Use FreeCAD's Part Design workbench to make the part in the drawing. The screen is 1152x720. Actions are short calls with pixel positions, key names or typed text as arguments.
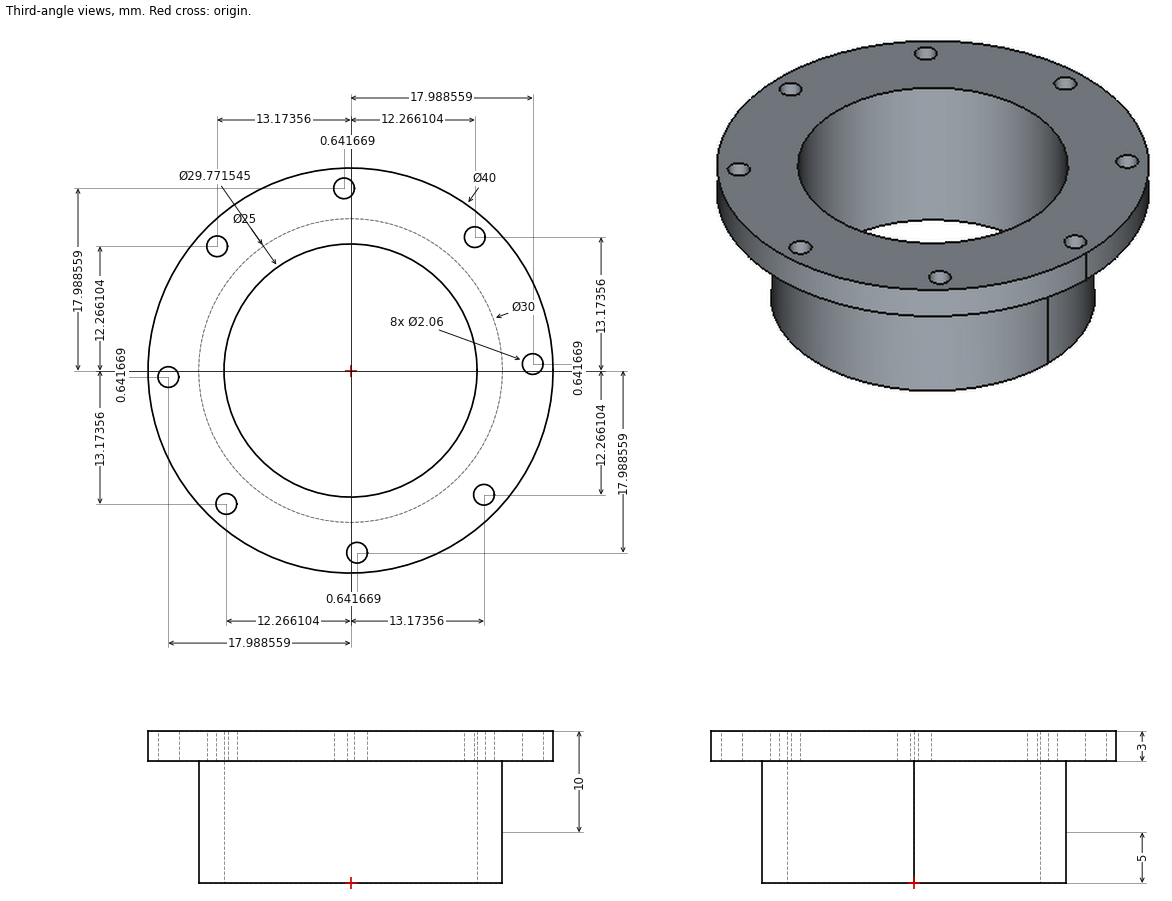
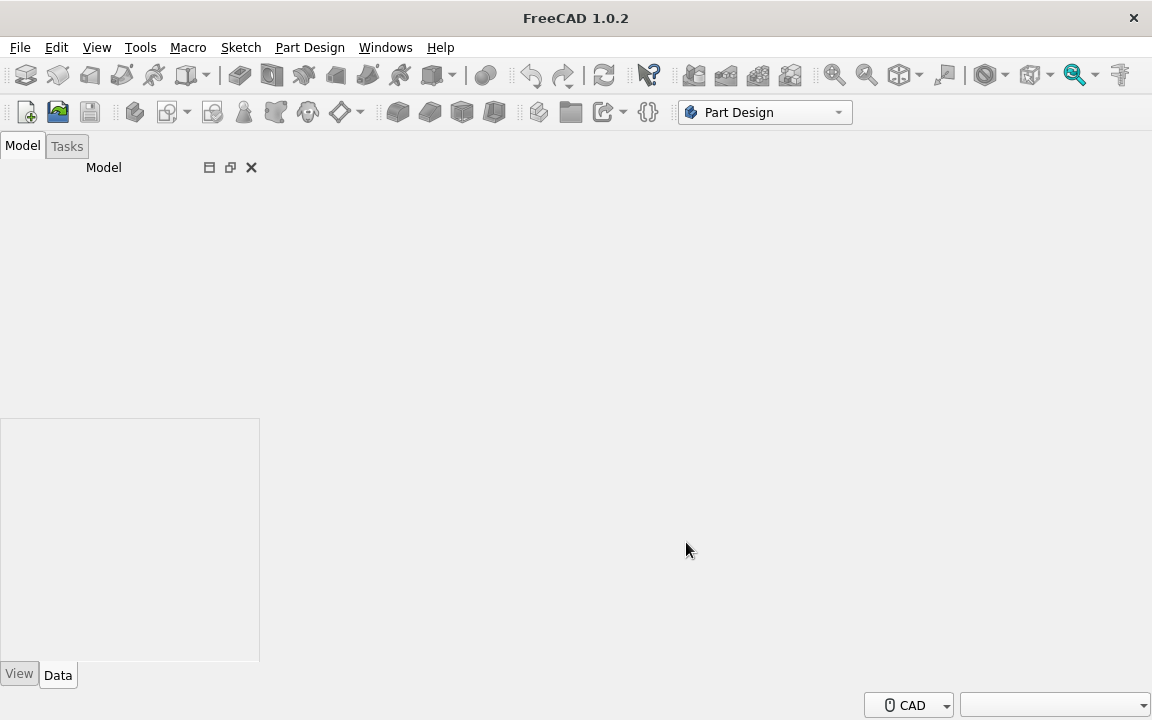
key(ctrl+n)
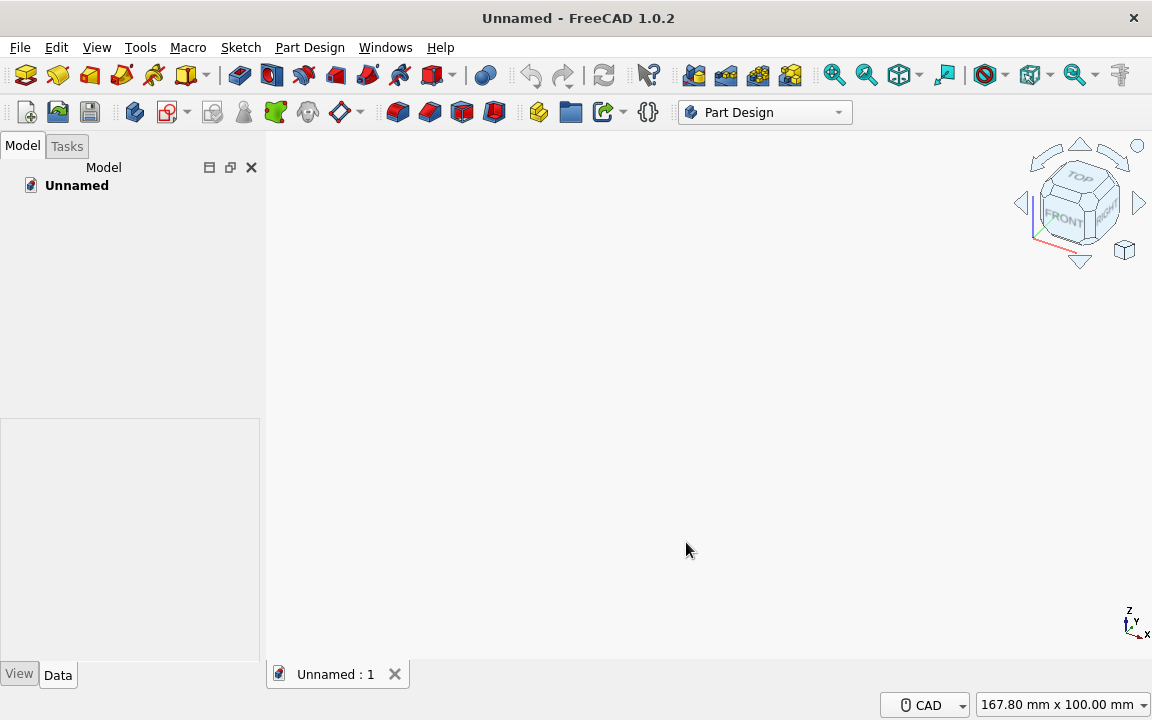
click(168, 112)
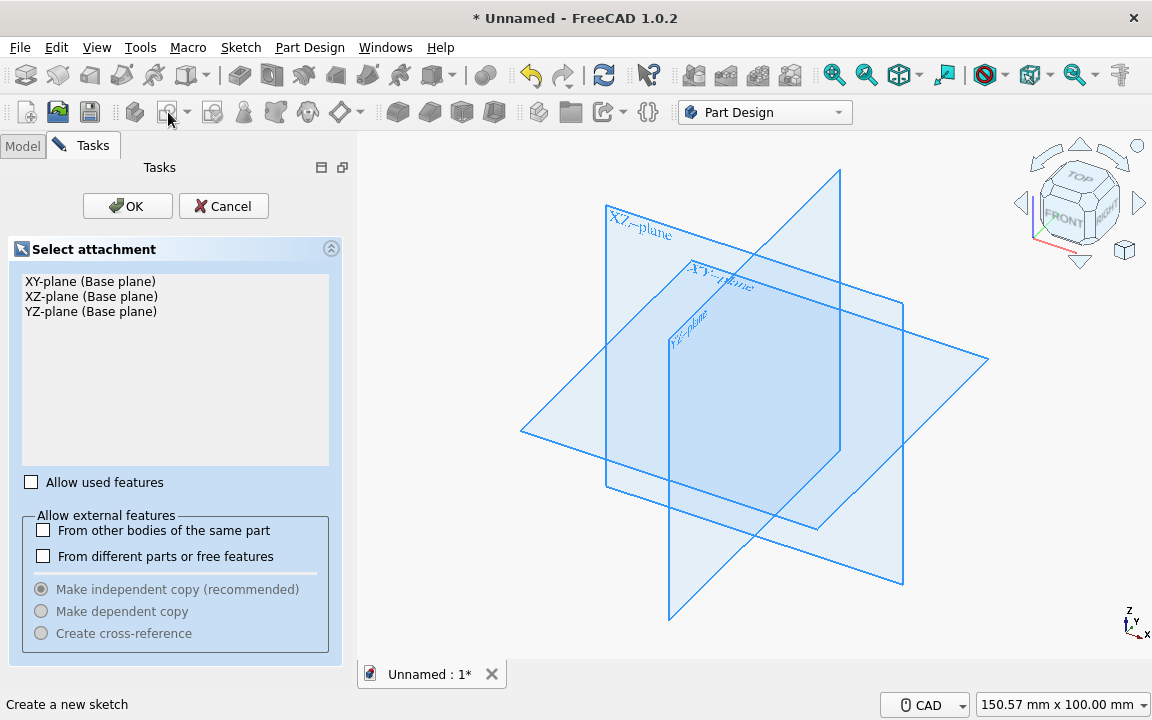
click(82, 282)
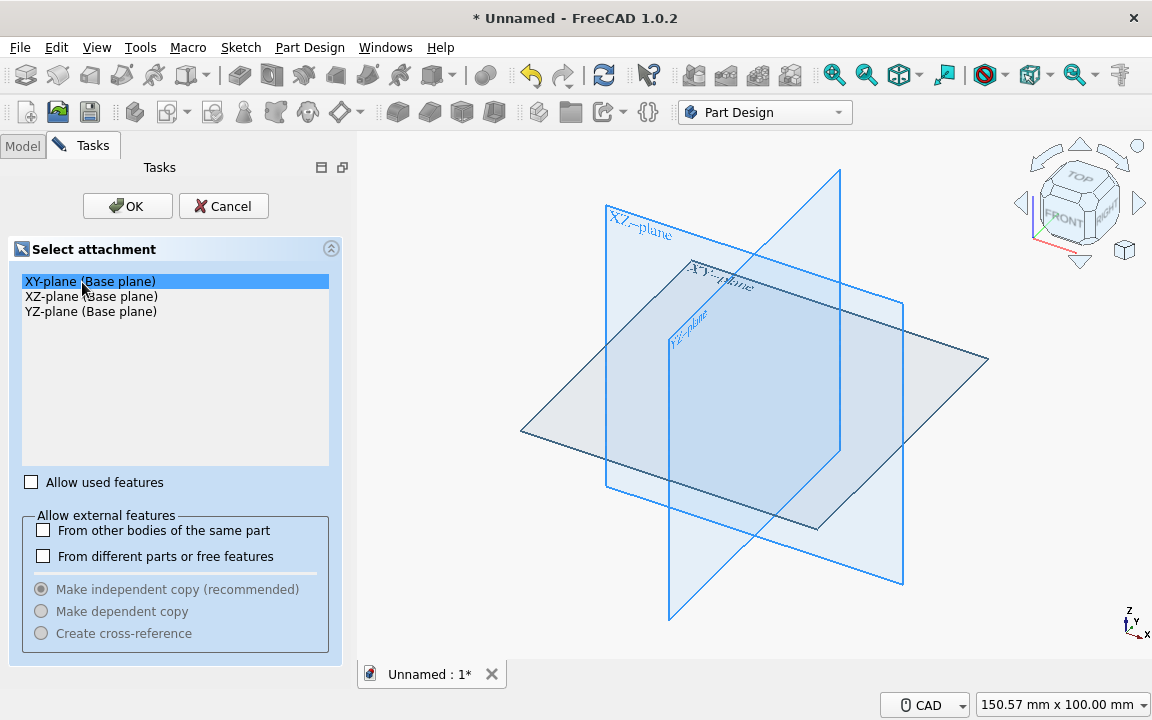
click(128, 206)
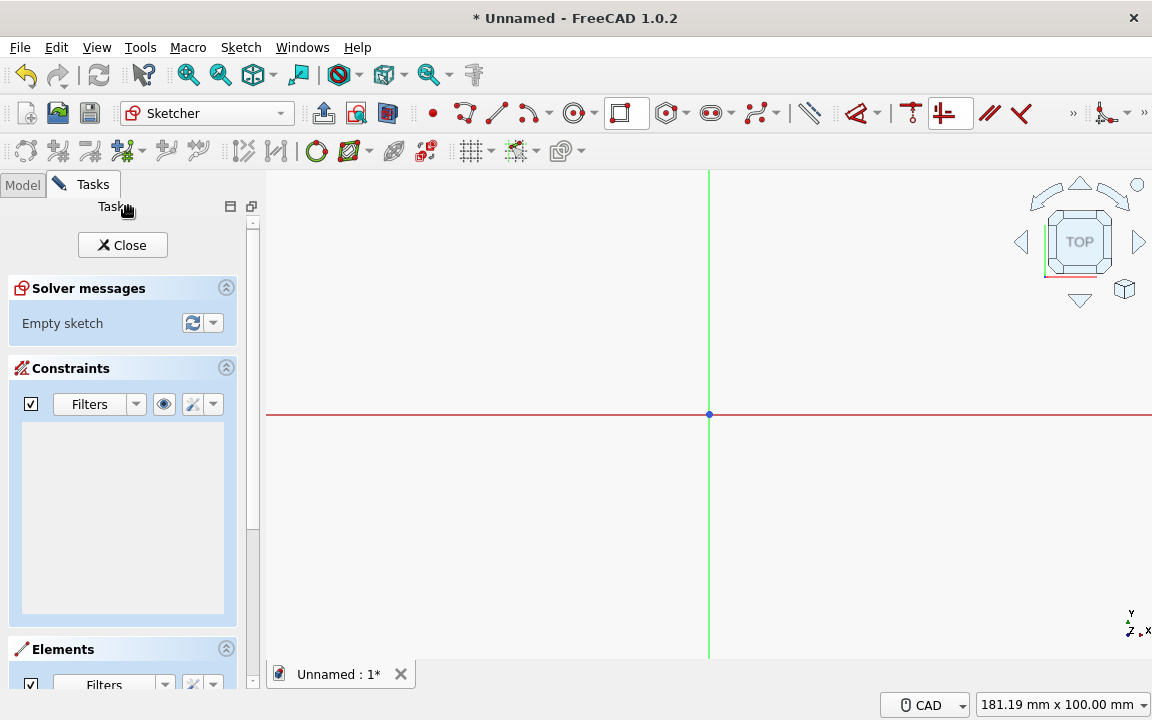
scroll(765, 414, up, 4)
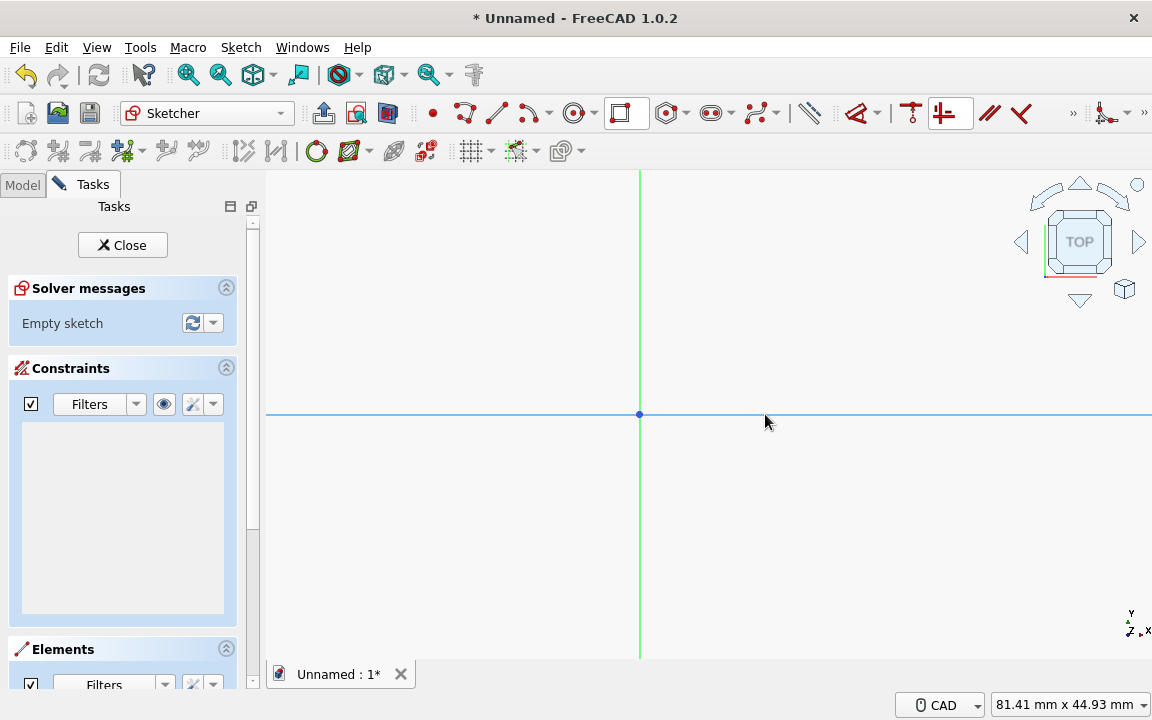
key(g)
key(c)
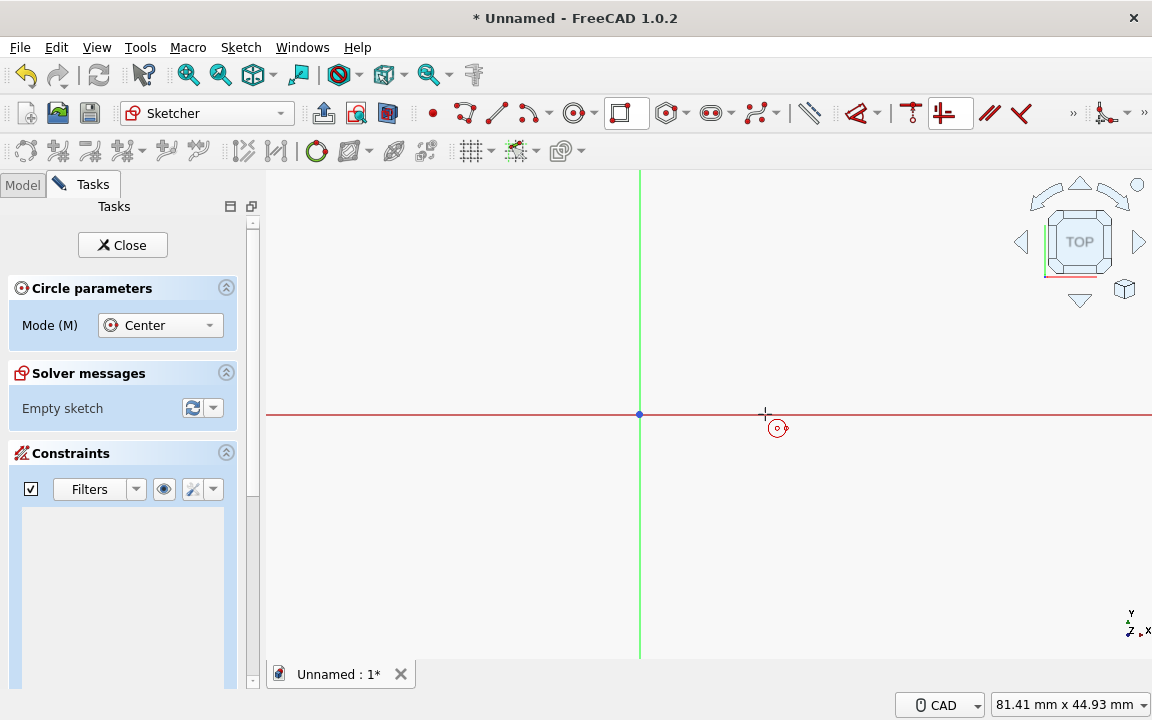
click(640, 414)
click(755, 299)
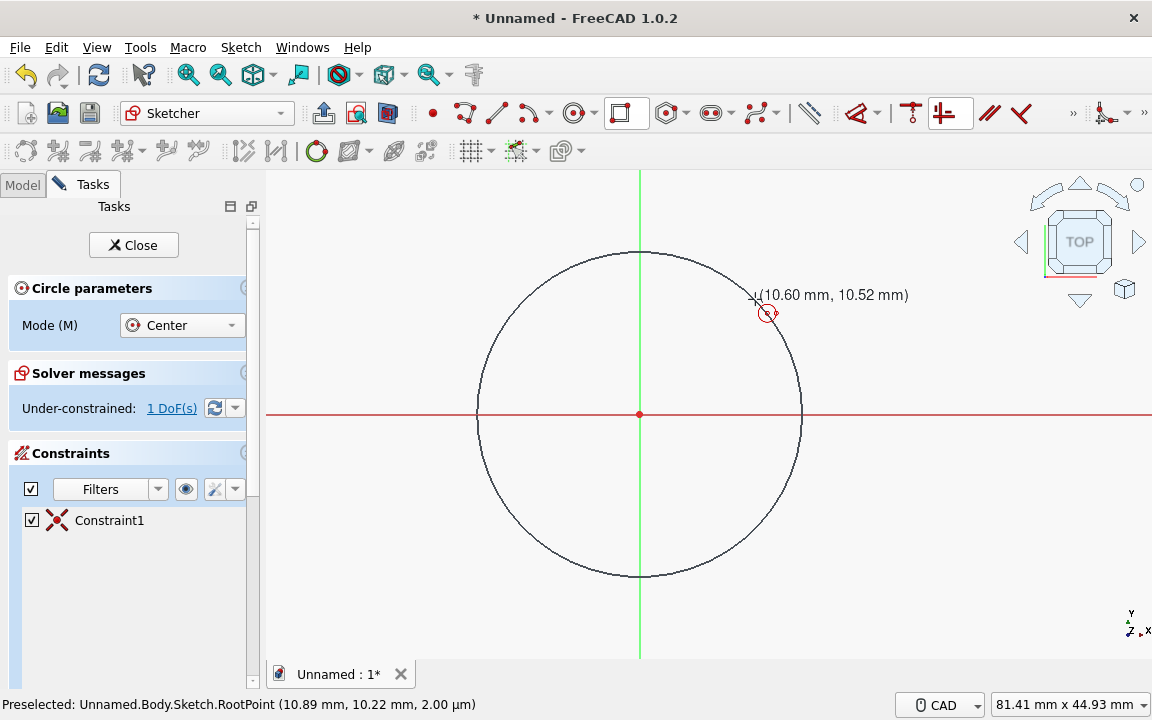
click(640, 414)
click(736, 318)
key(Escape)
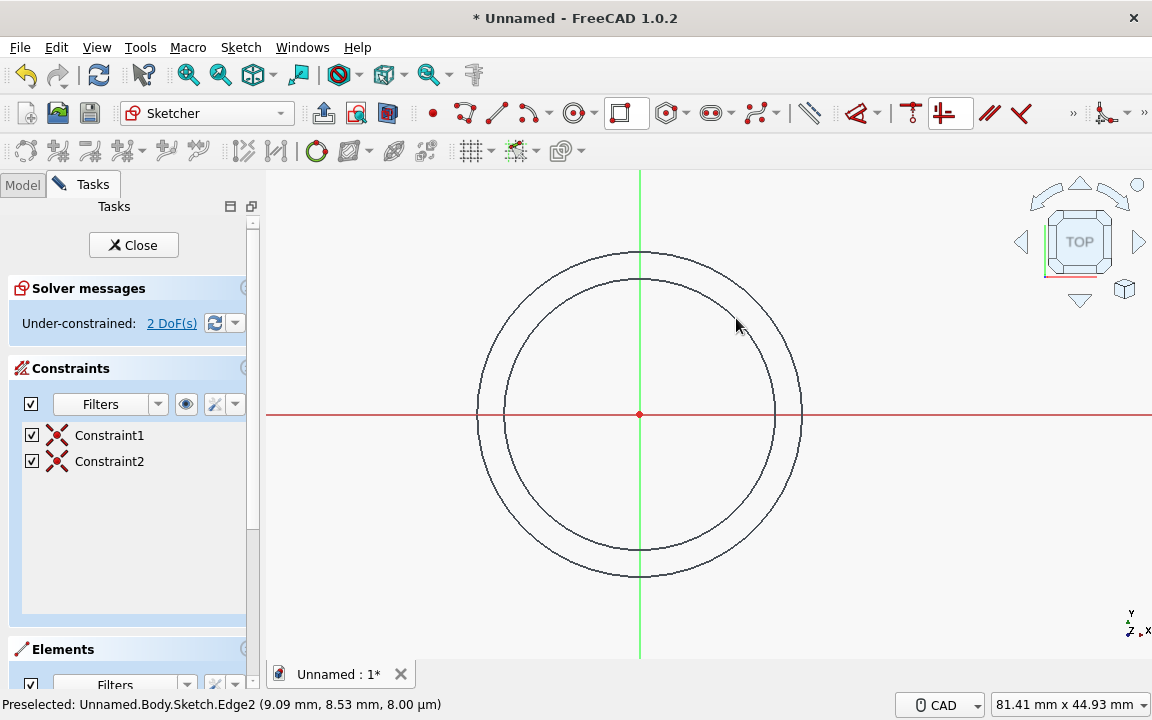
click(856, 114)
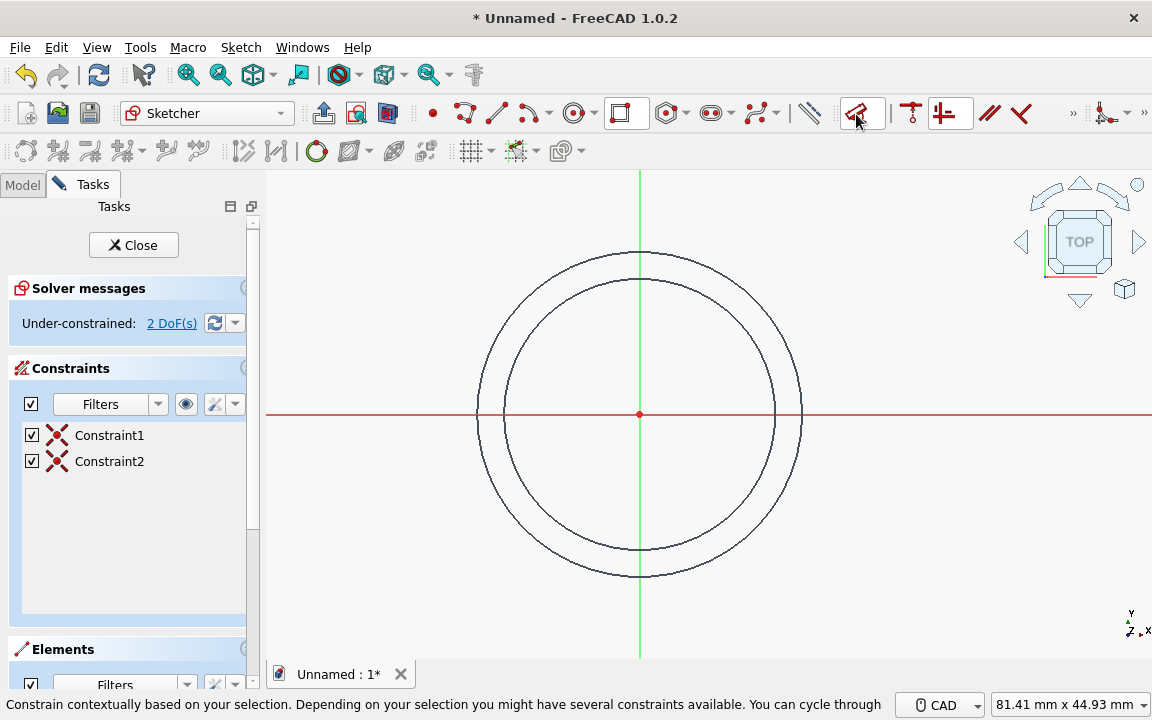
click(754, 299)
click(777, 276)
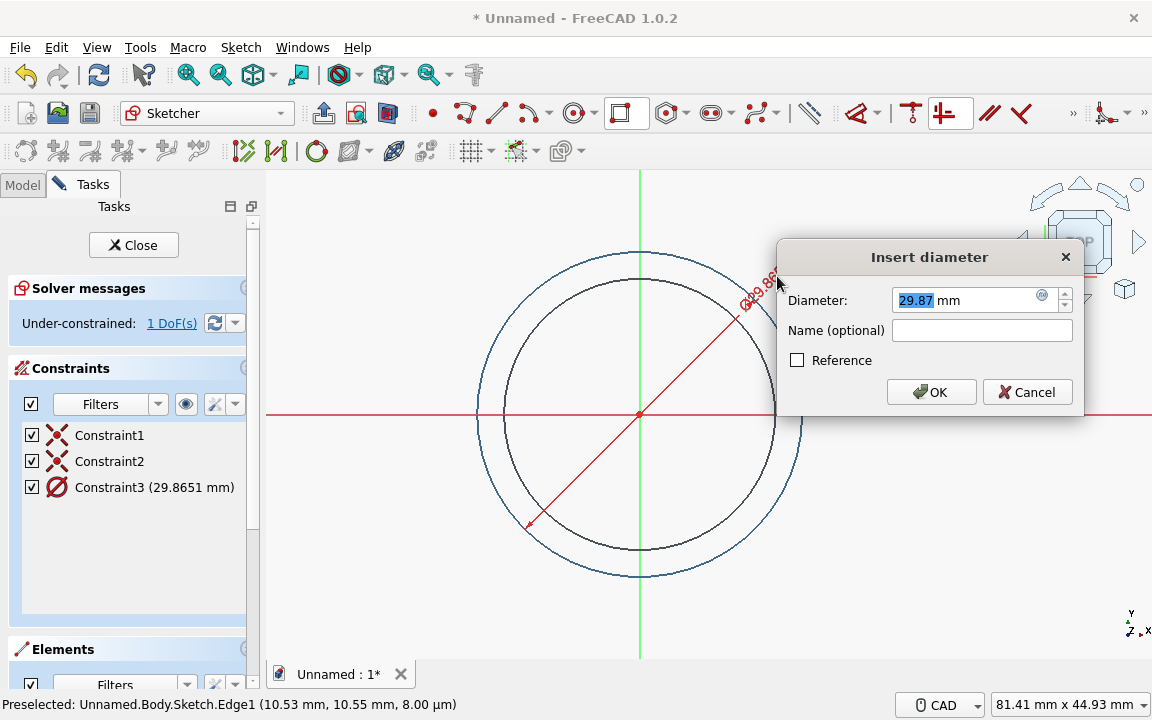
text(30)
key(Return)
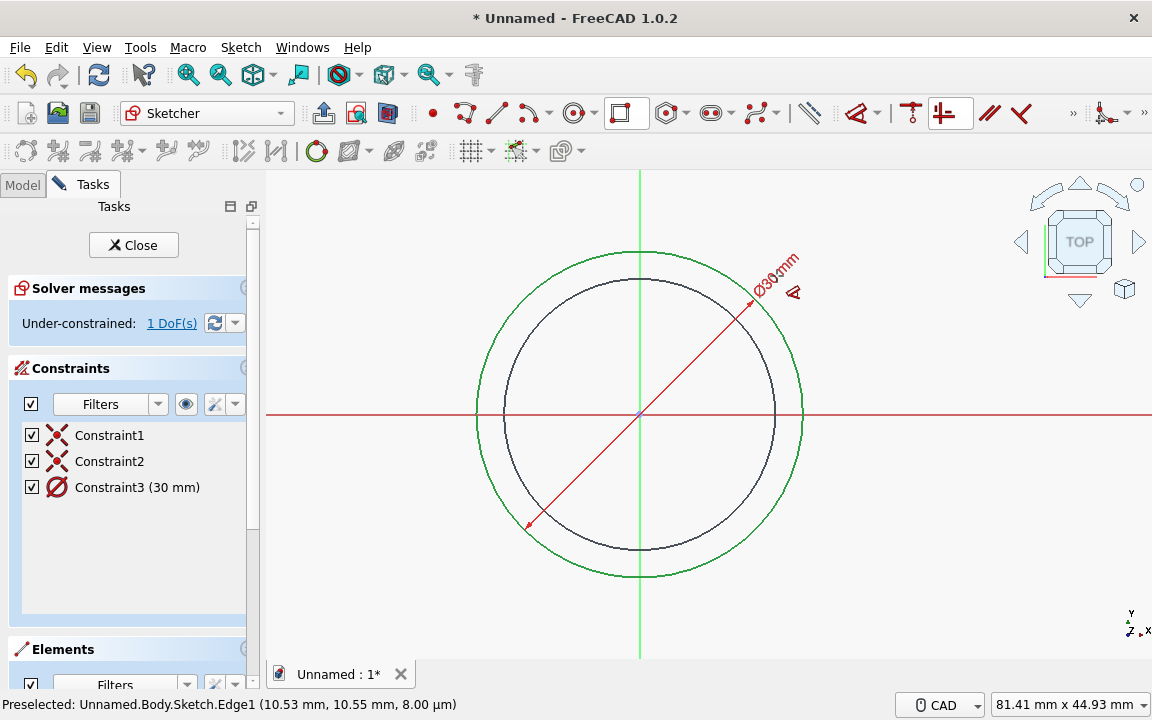
click(735, 318)
click(822, 360)